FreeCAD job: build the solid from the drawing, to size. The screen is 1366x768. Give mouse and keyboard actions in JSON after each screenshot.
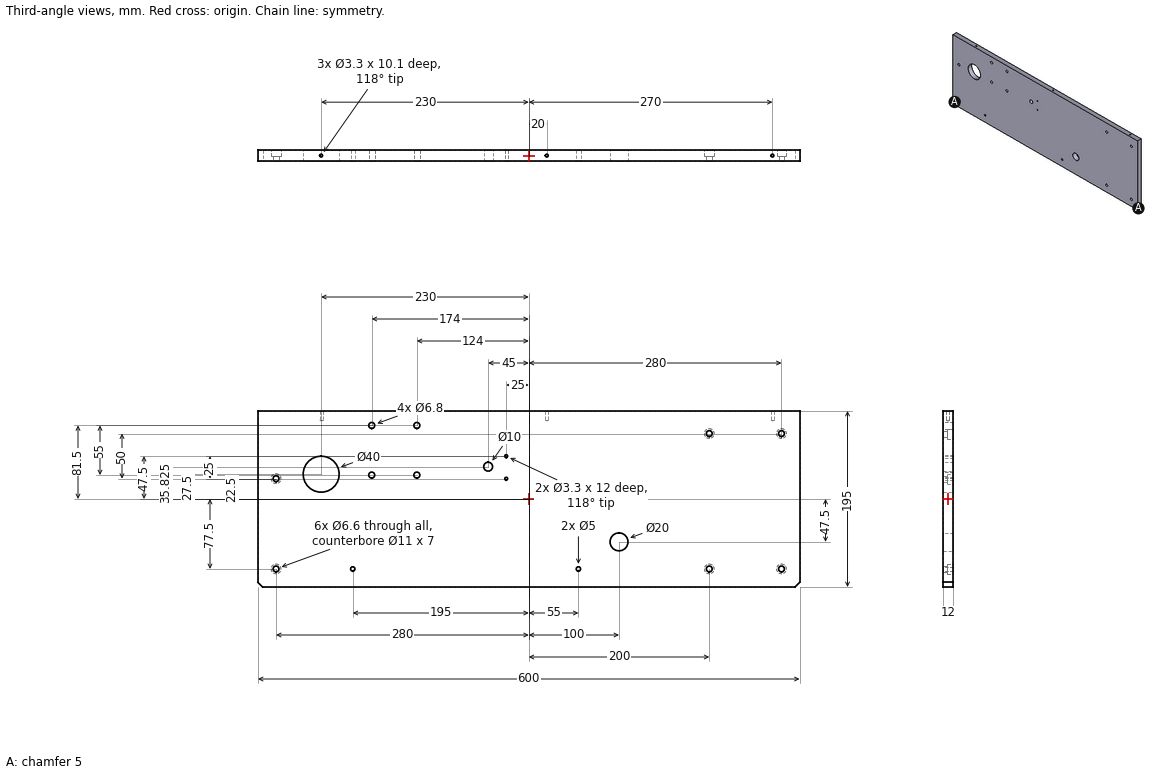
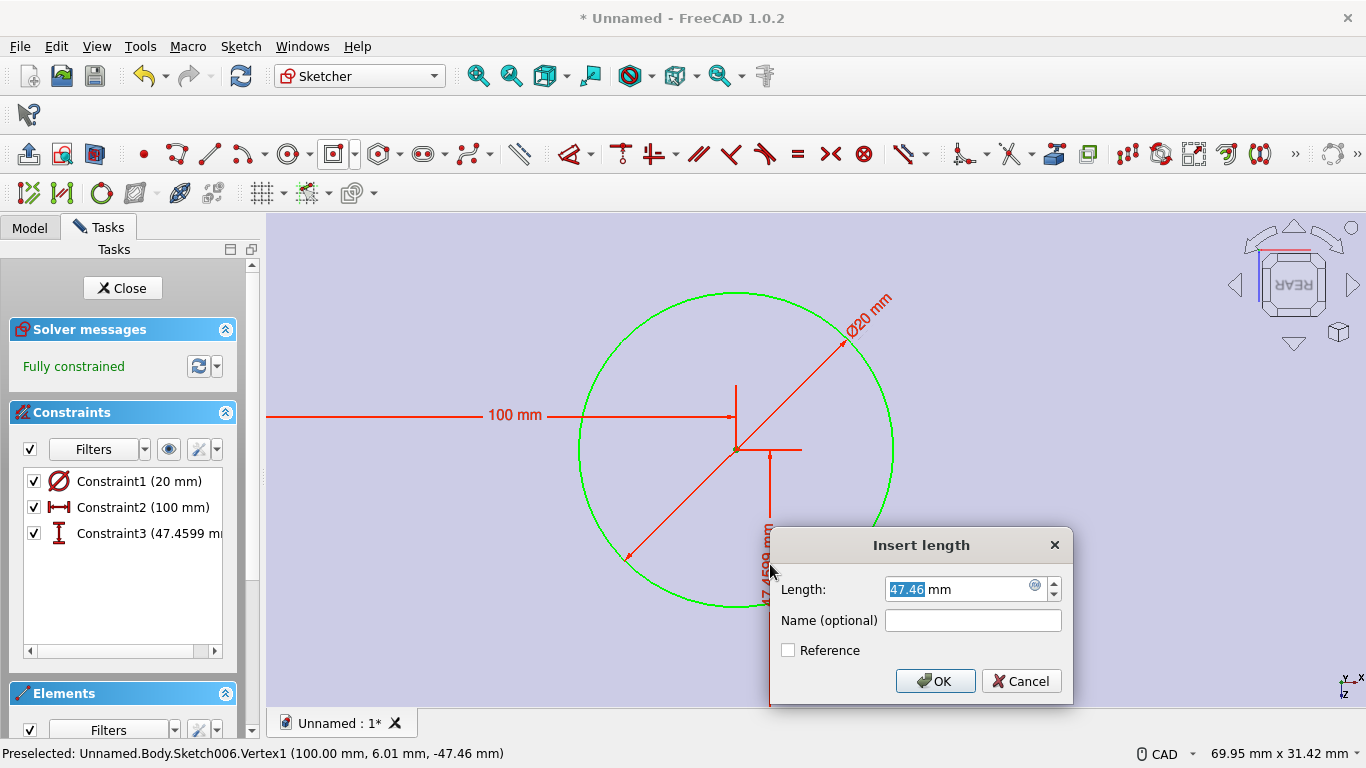
{"action": "type", "text": "47.5"}
{"action": "key", "text": "Return"}
{"action": "key", "text": "Escape"}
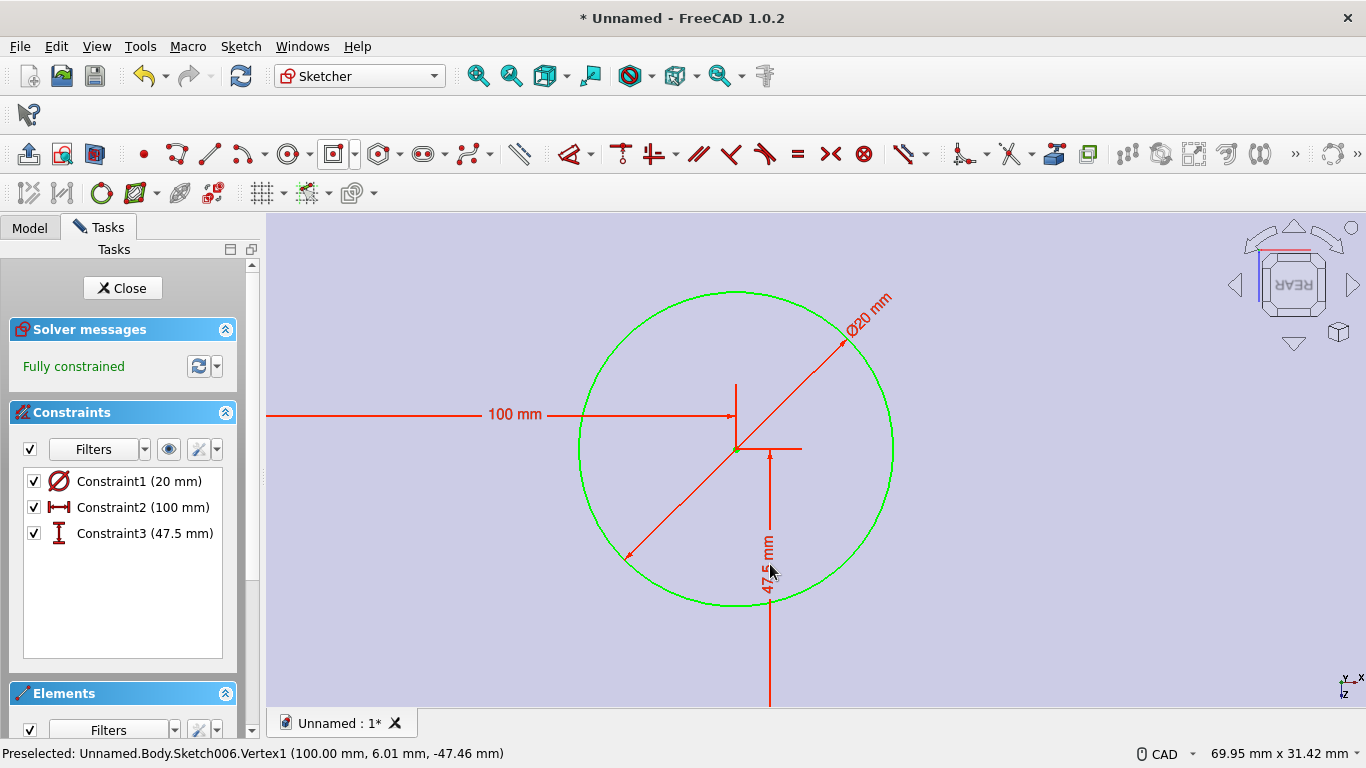
{"action": "left_click", "coordinate": [123, 288]}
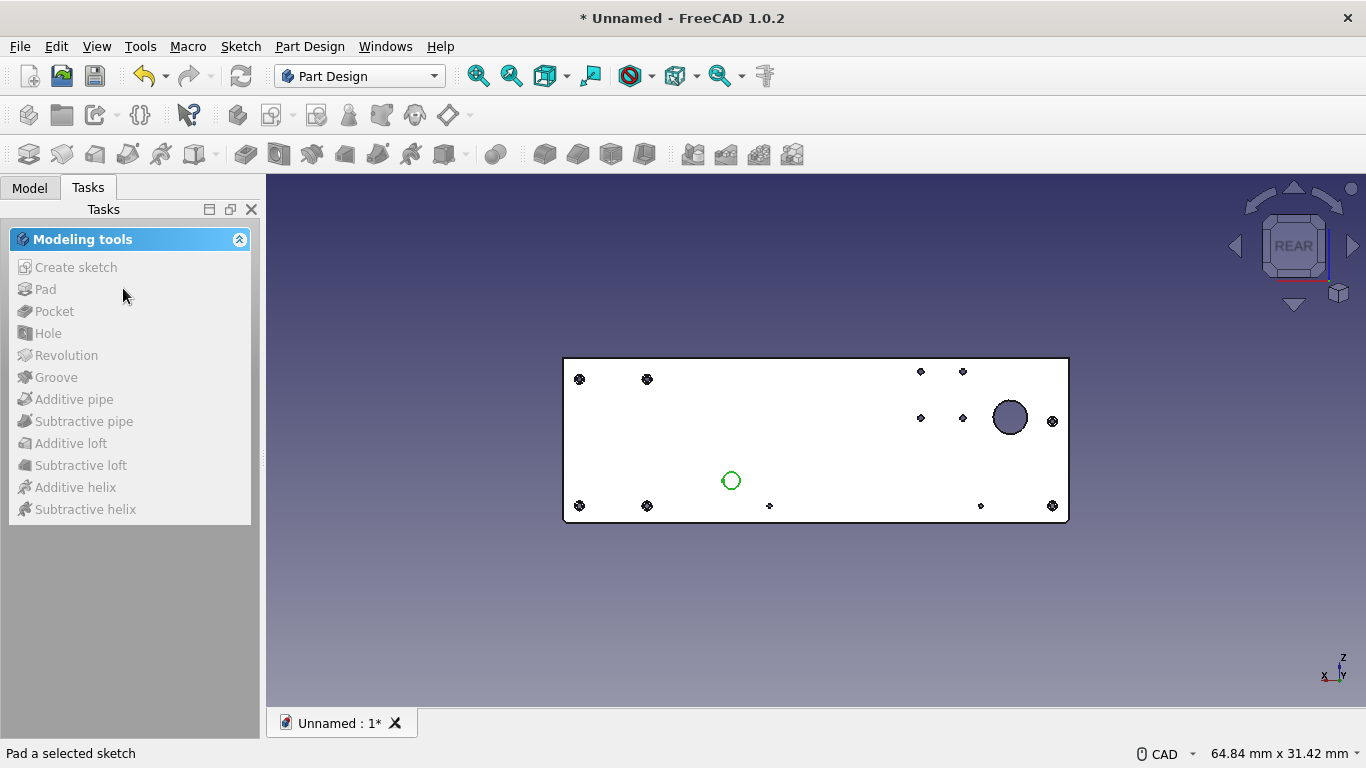
{"action": "left_click", "coordinate": [246, 154]}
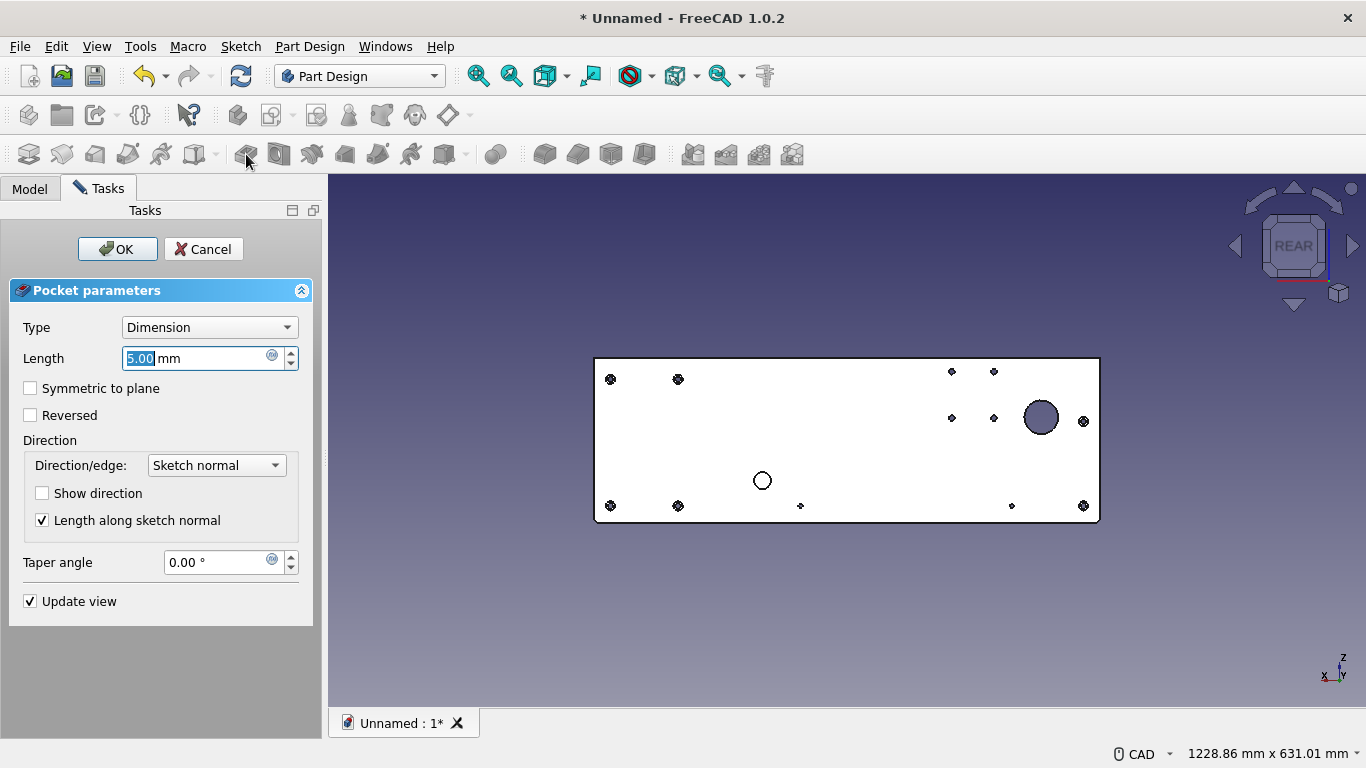
{"action": "left_click", "coordinate": [210, 328]}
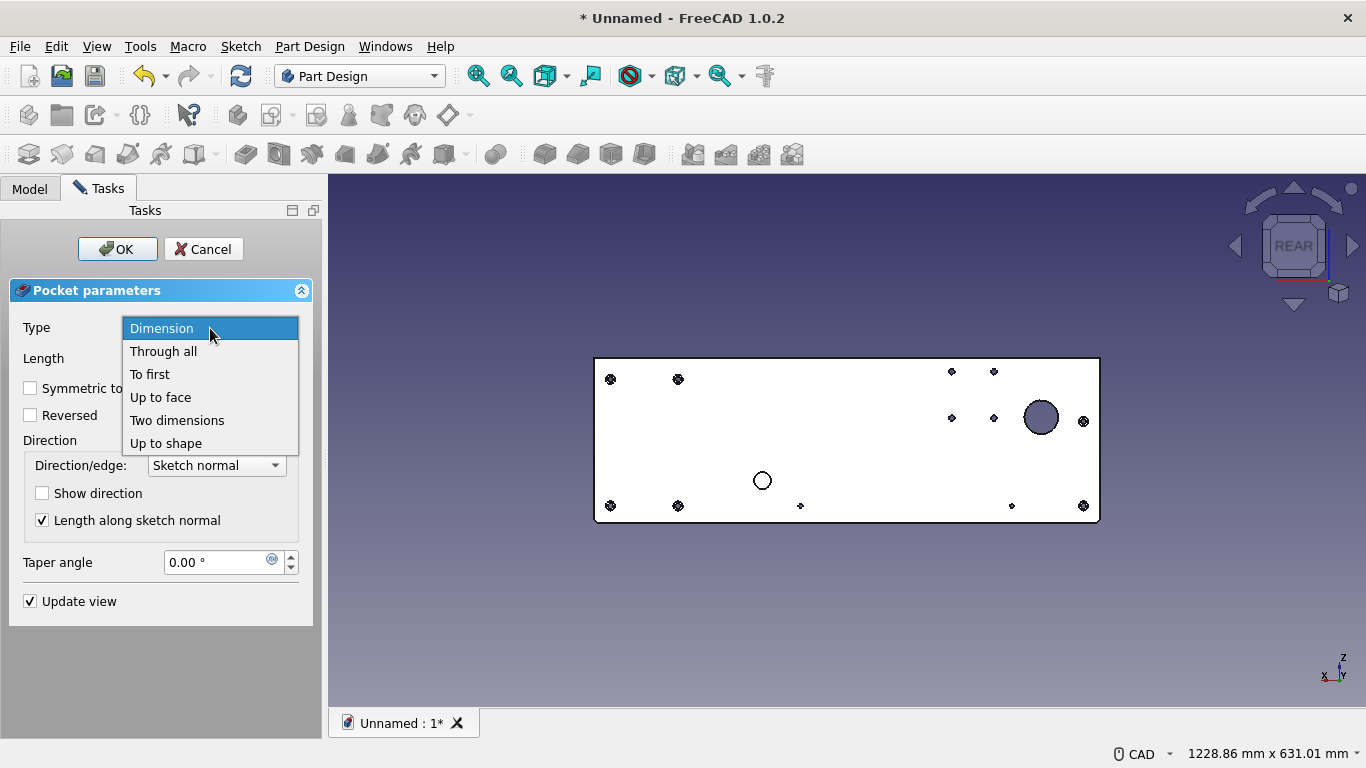
{"action": "left_click", "coordinate": [208, 352]}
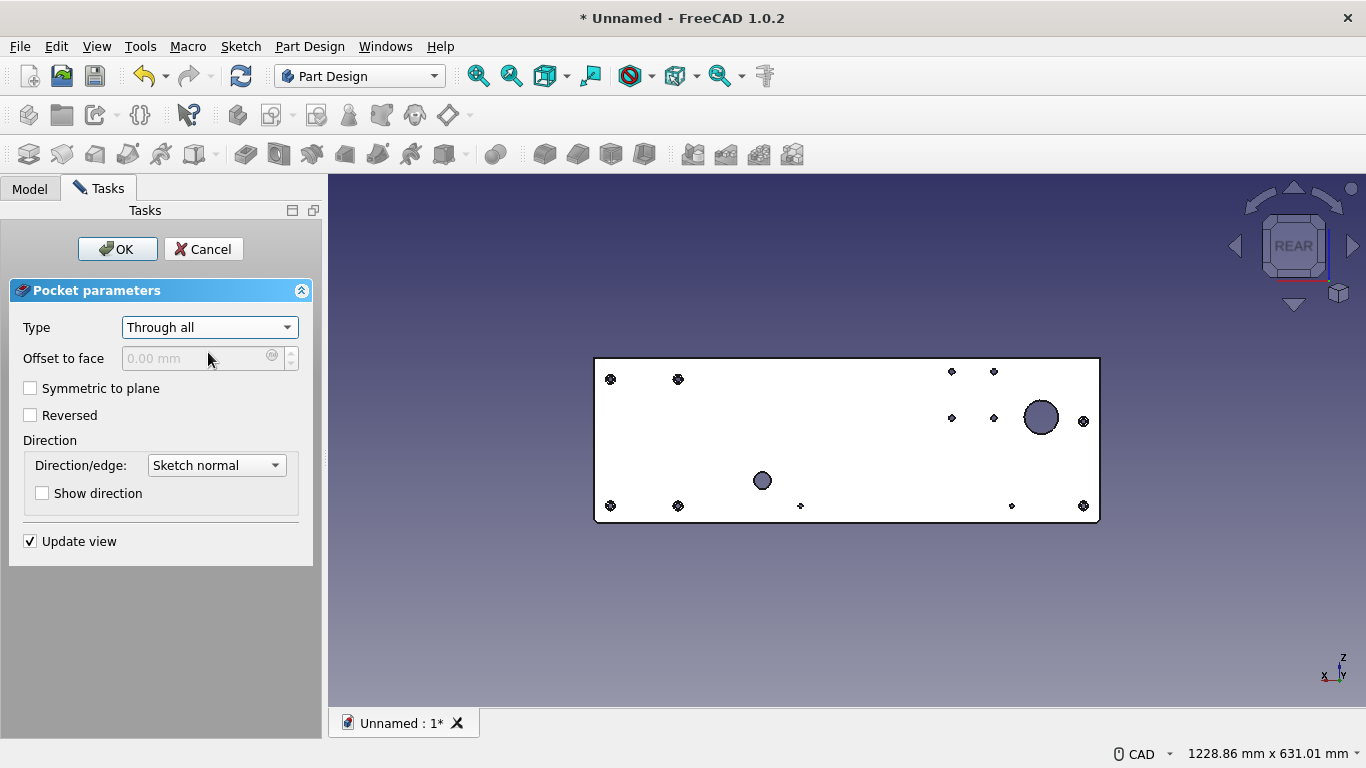
{"action": "left_click", "coordinate": [118, 249]}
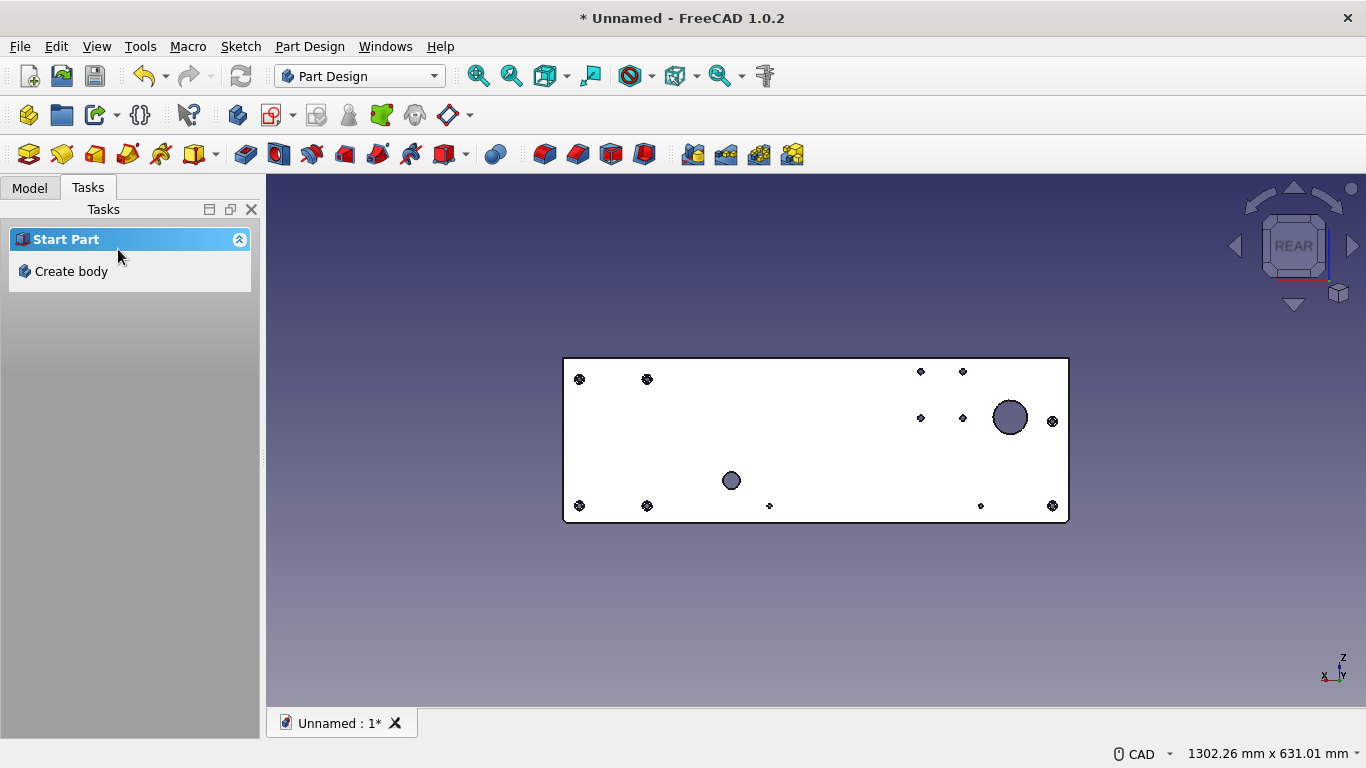
{"action": "left_click", "coordinate": [816, 439]}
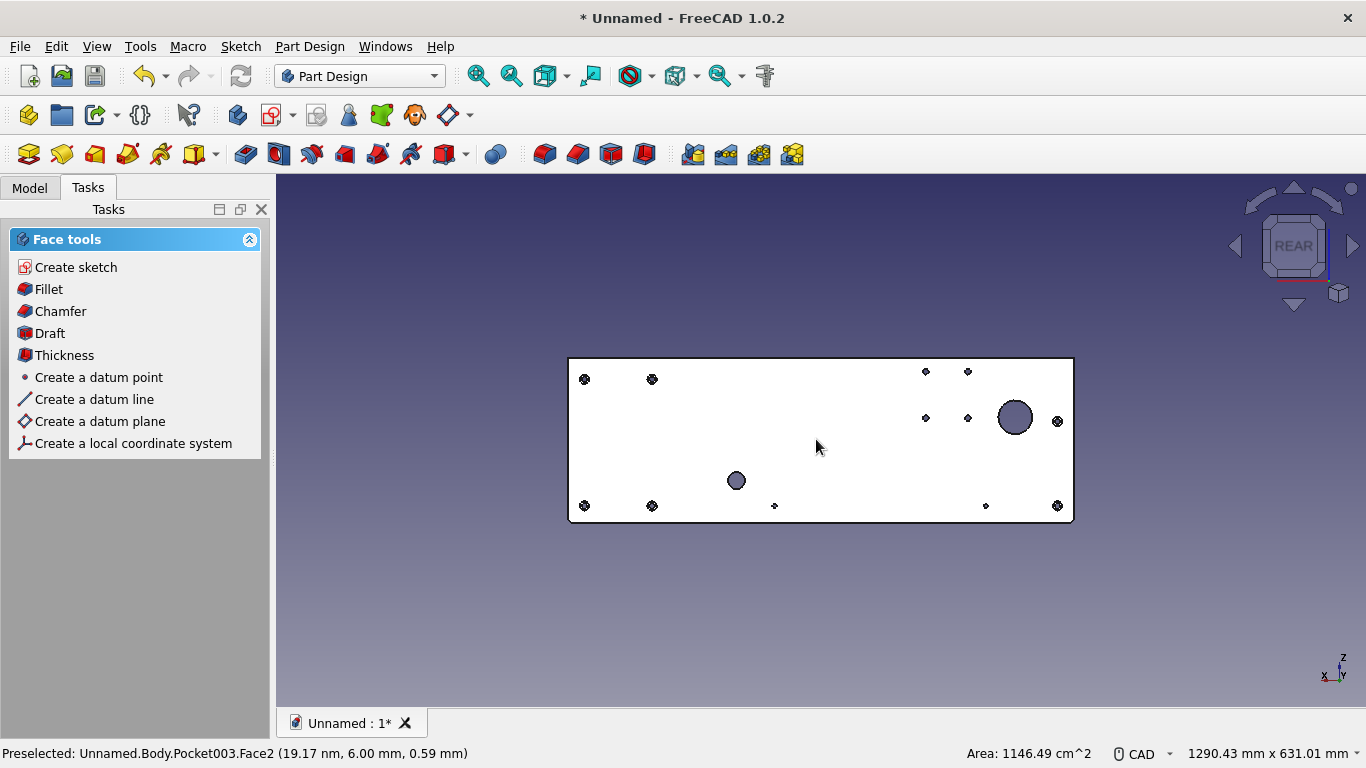
{"action": "left_click", "coordinate": [270, 116]}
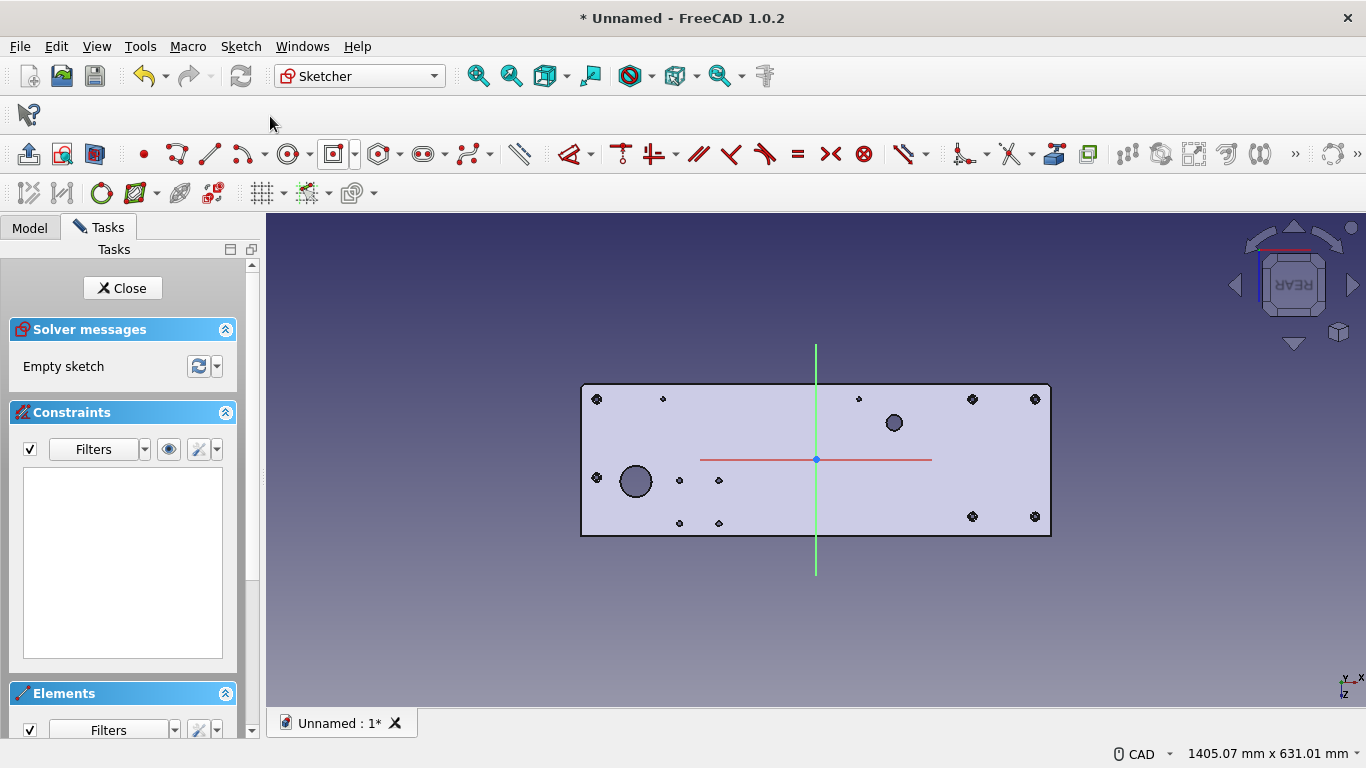
{"action": "scroll", "coordinate": [815, 482], "scroll_direction": "up", "scroll_amount": 10}